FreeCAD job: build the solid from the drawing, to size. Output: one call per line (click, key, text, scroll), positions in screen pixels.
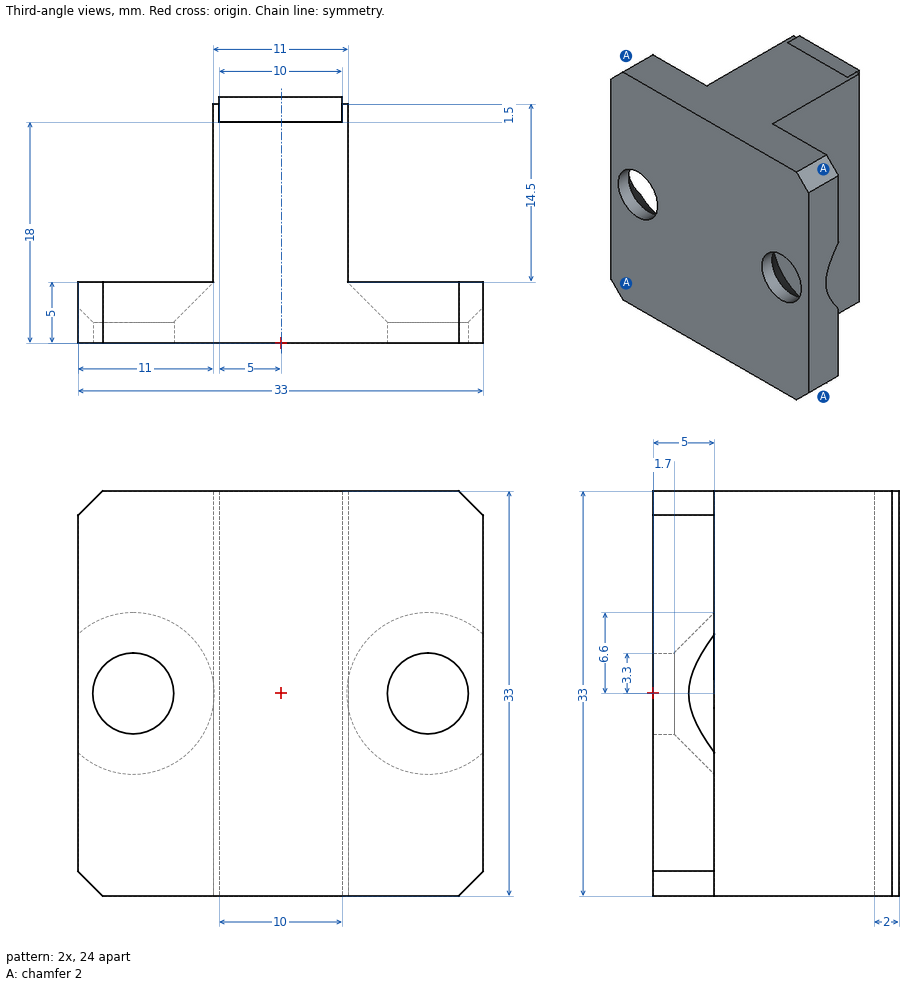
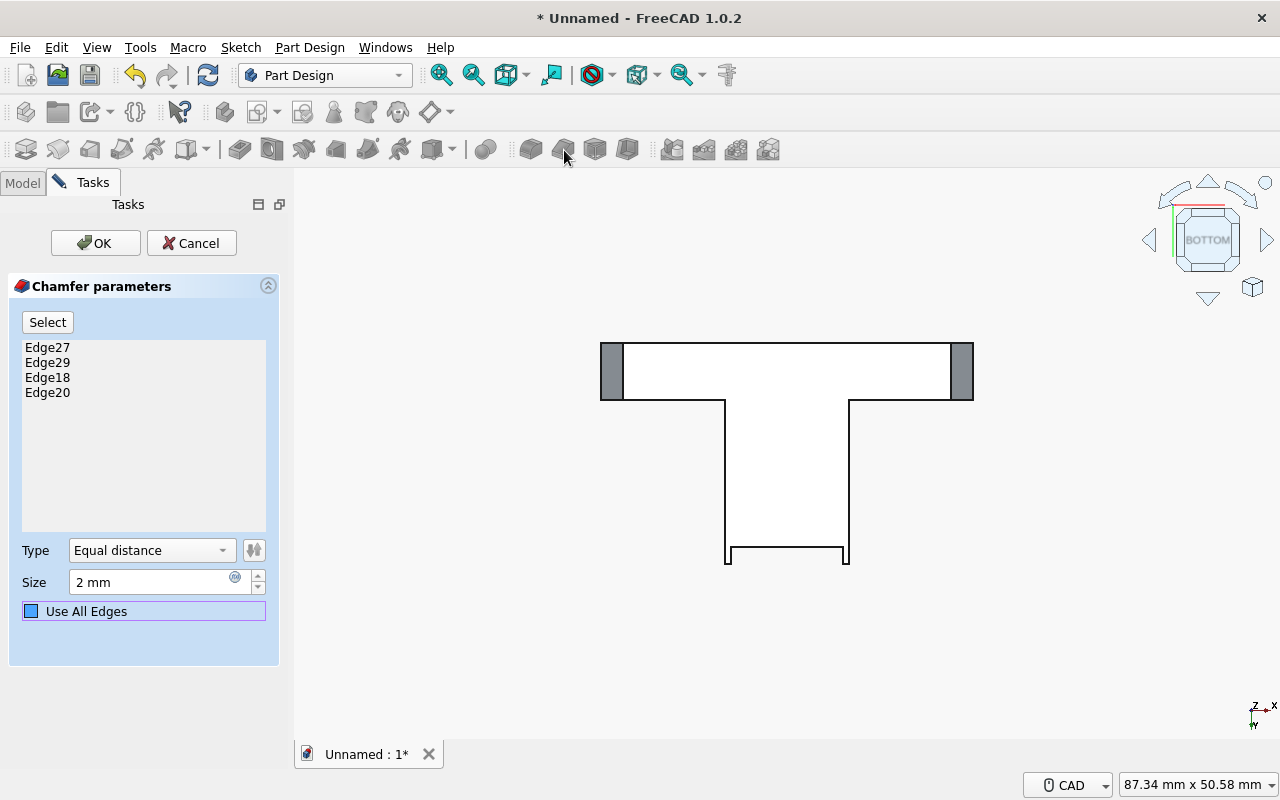
click(96, 243)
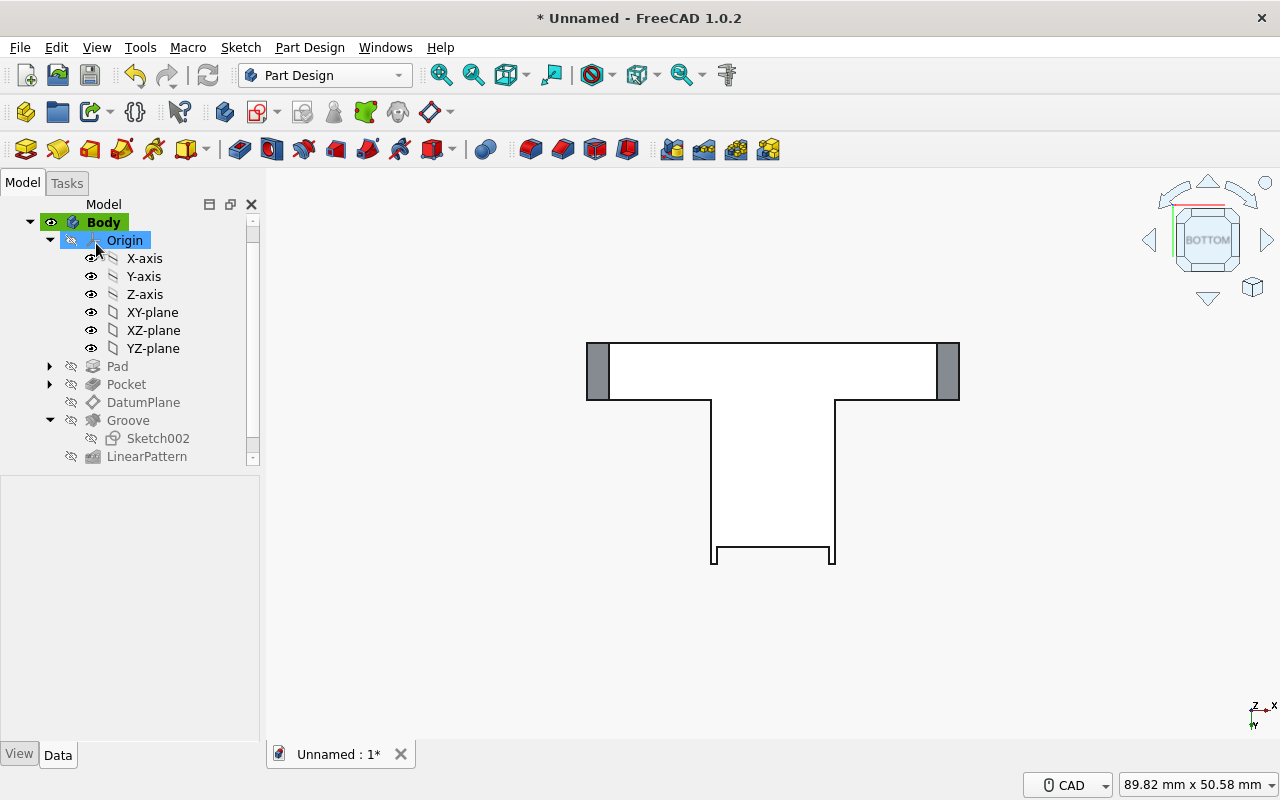
click(442, 76)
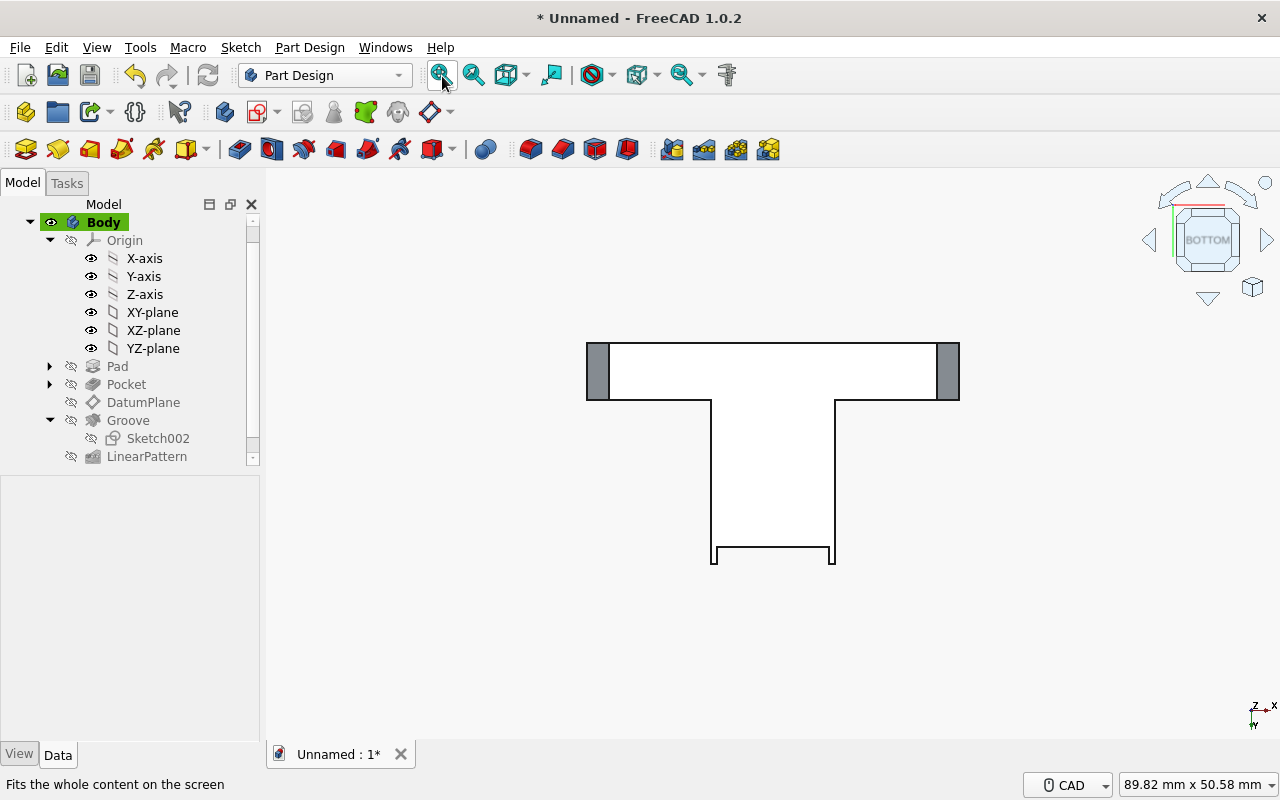
click(226, 112)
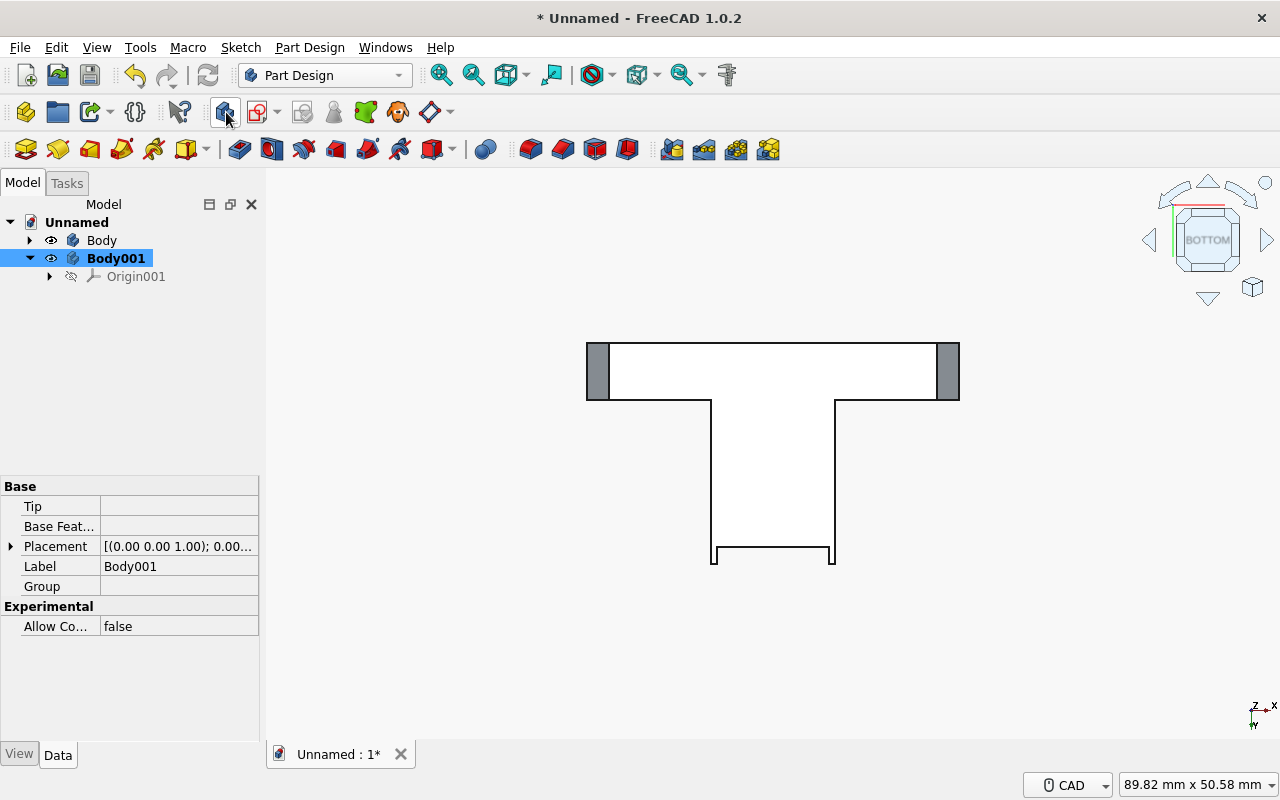
click(50, 276)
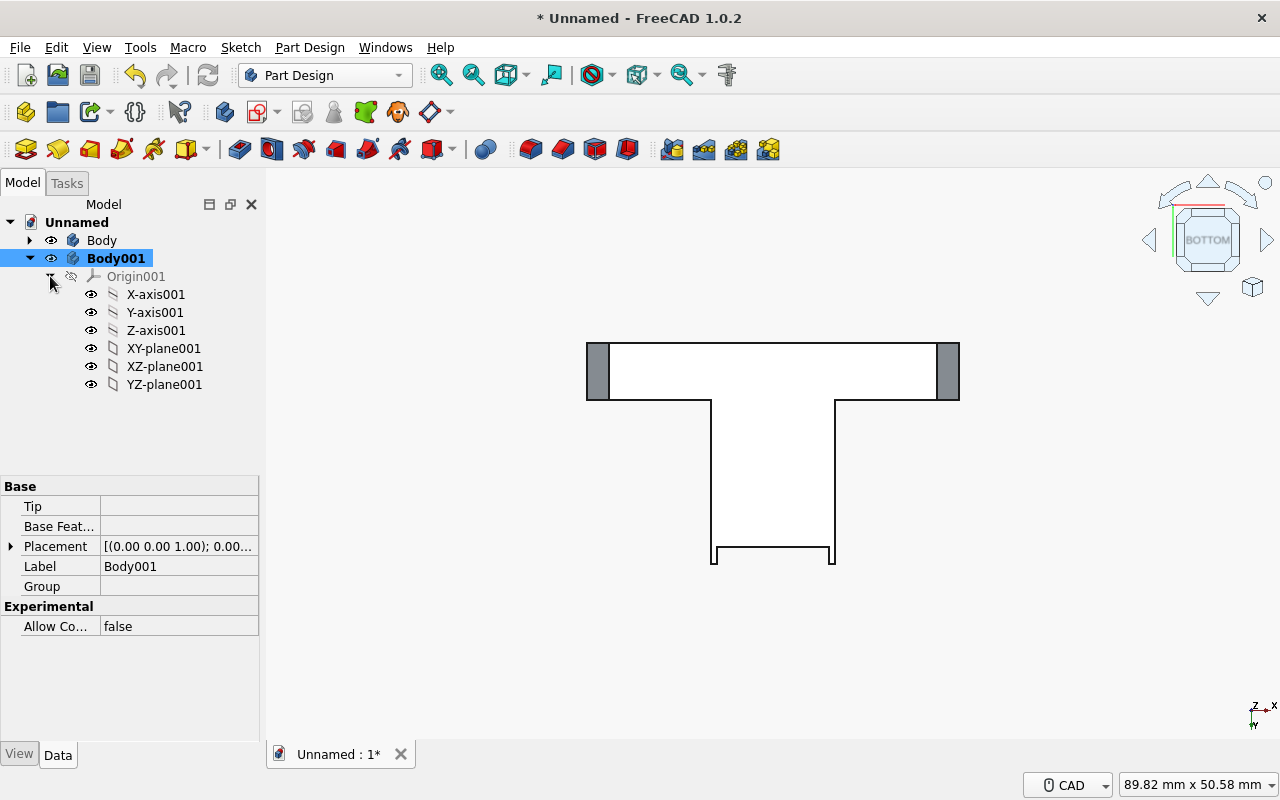
click(136, 366)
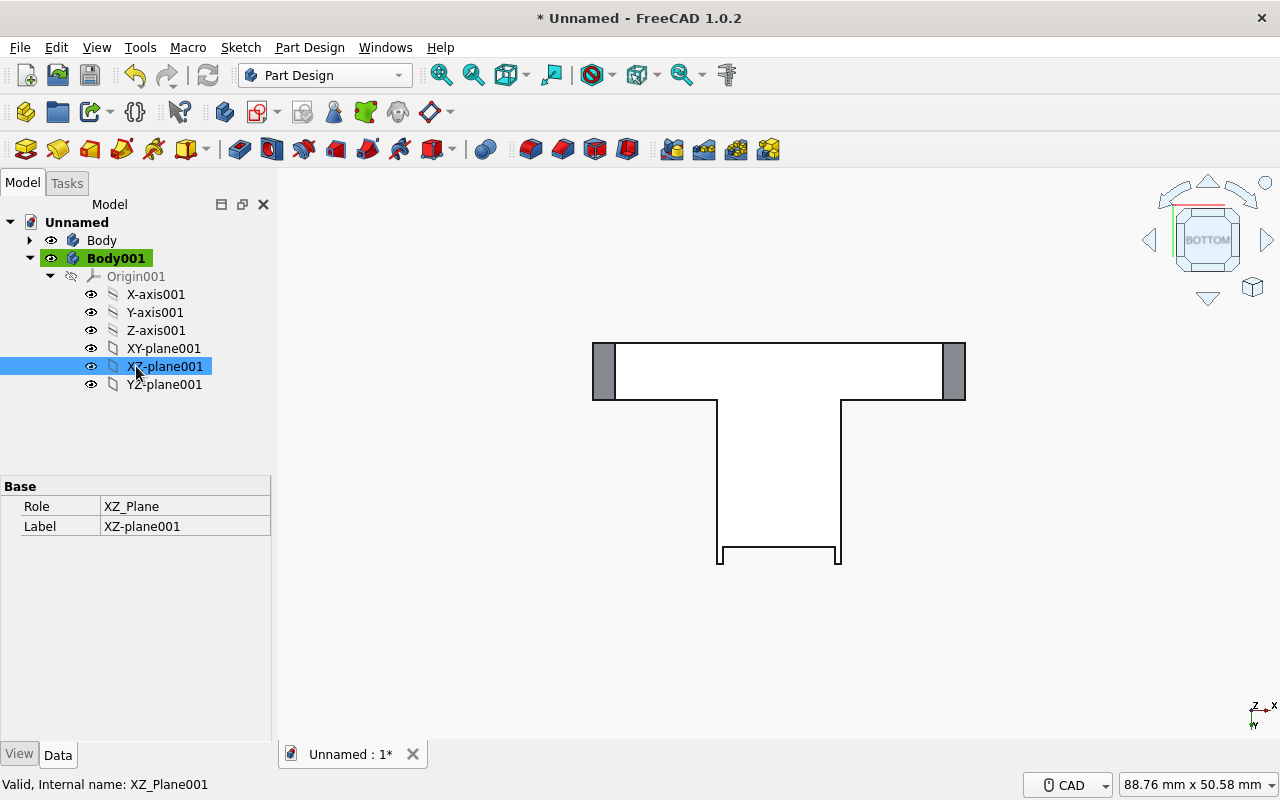
click(430, 112)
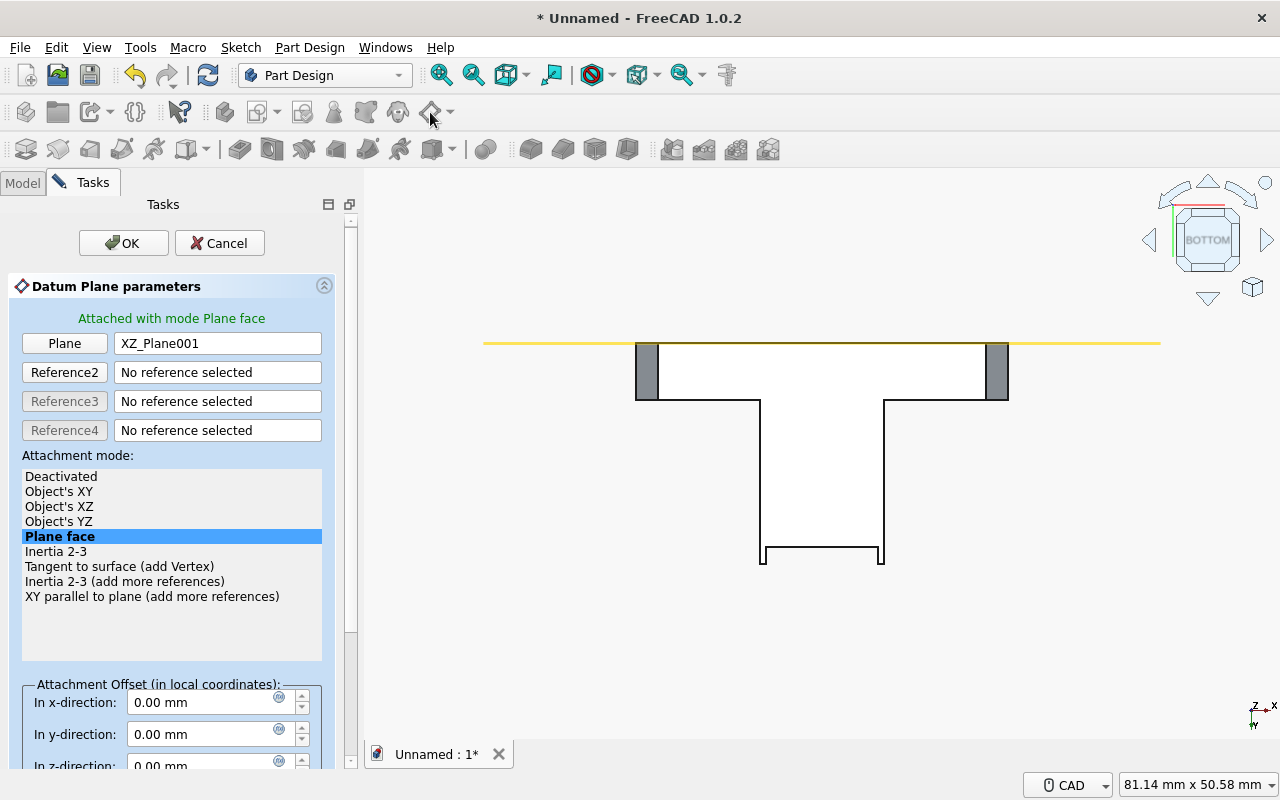
scroll(351, 491, down, 2)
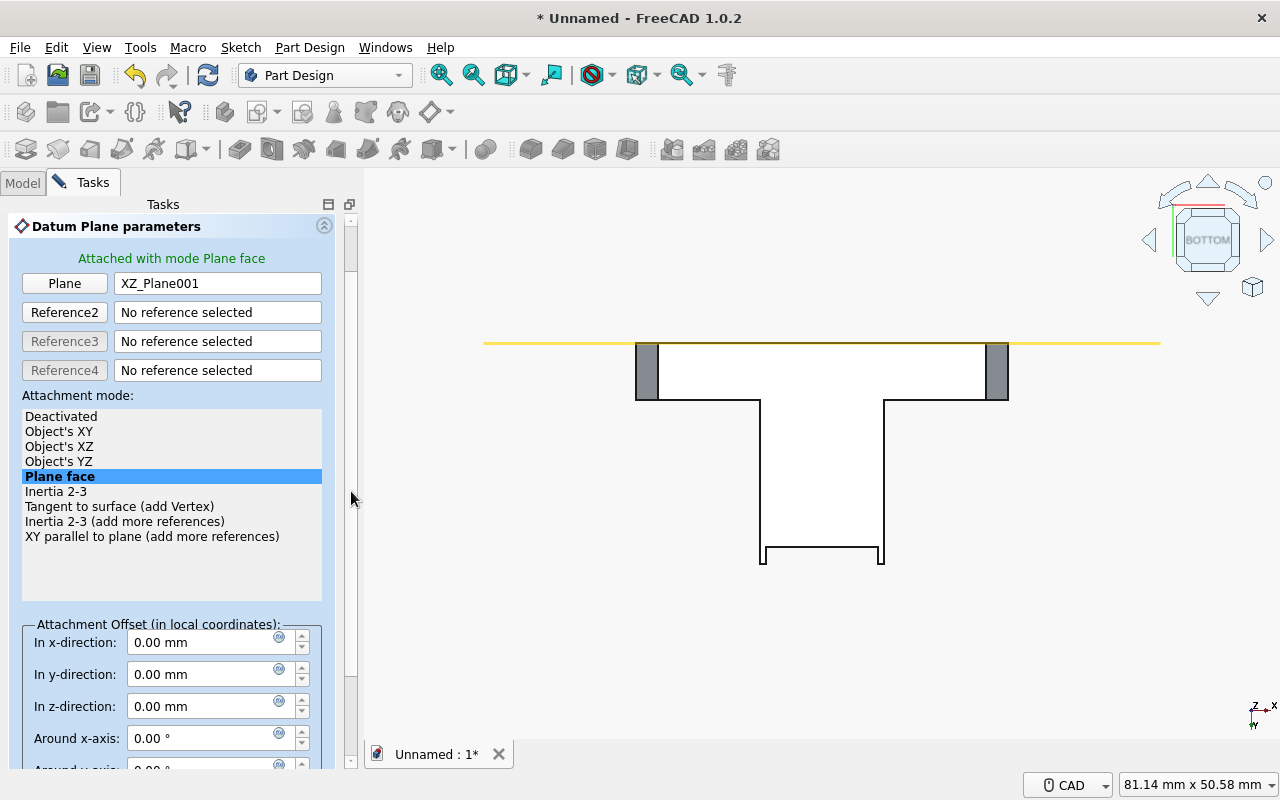
triple_click(210, 646)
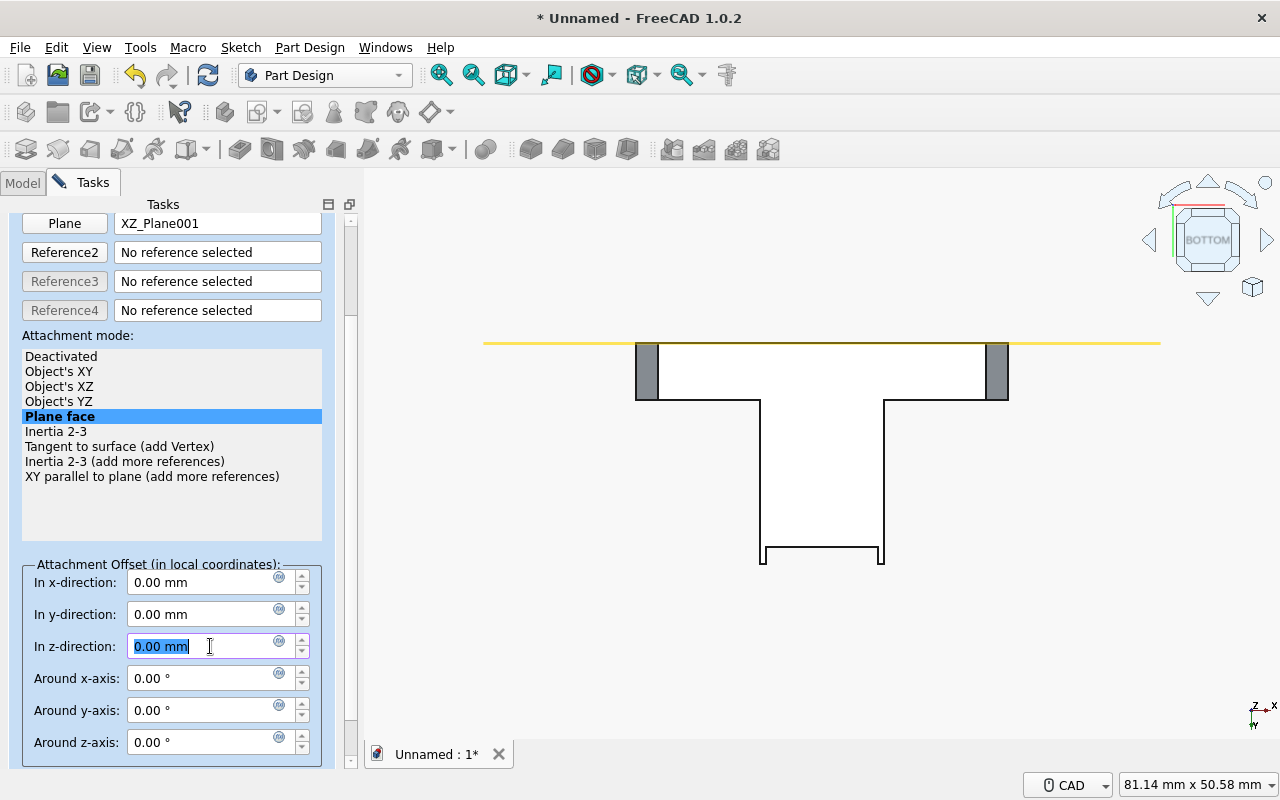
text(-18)
key(Tab)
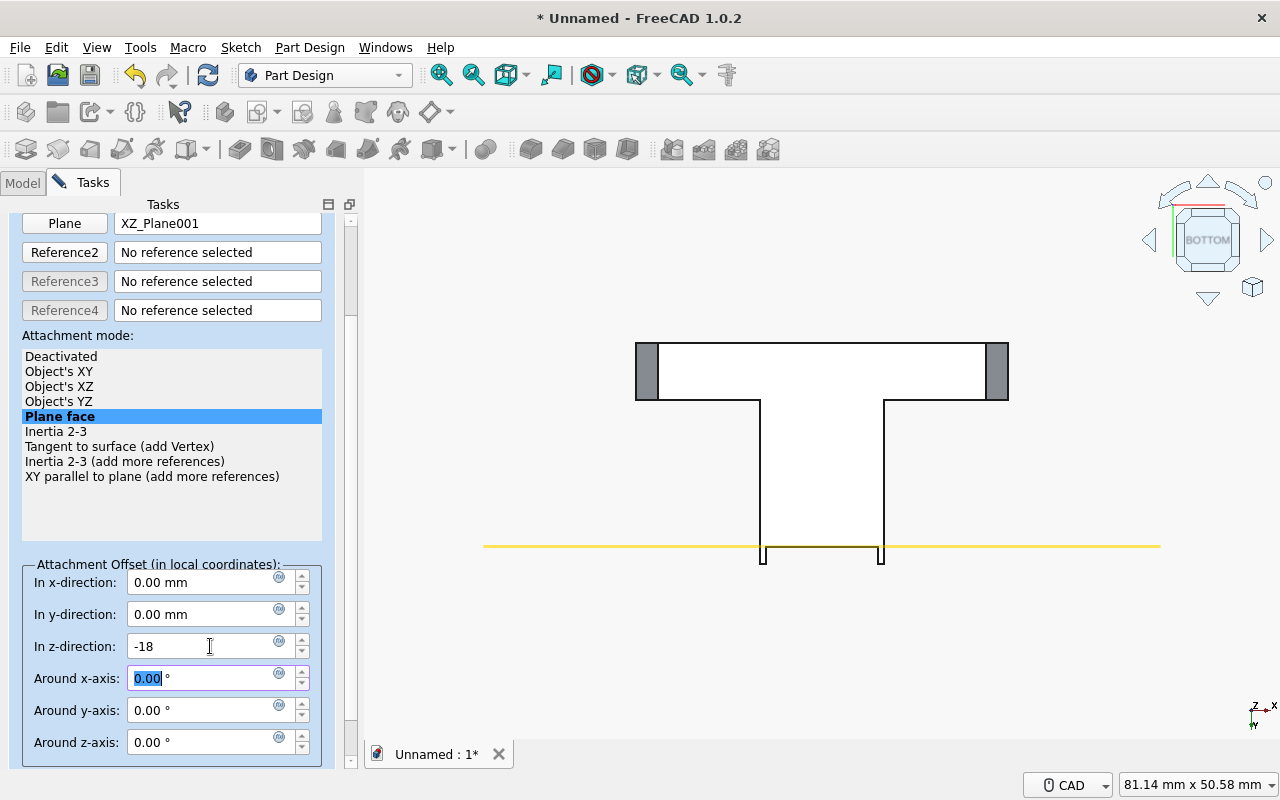
scroll(351, 491, up, 3)